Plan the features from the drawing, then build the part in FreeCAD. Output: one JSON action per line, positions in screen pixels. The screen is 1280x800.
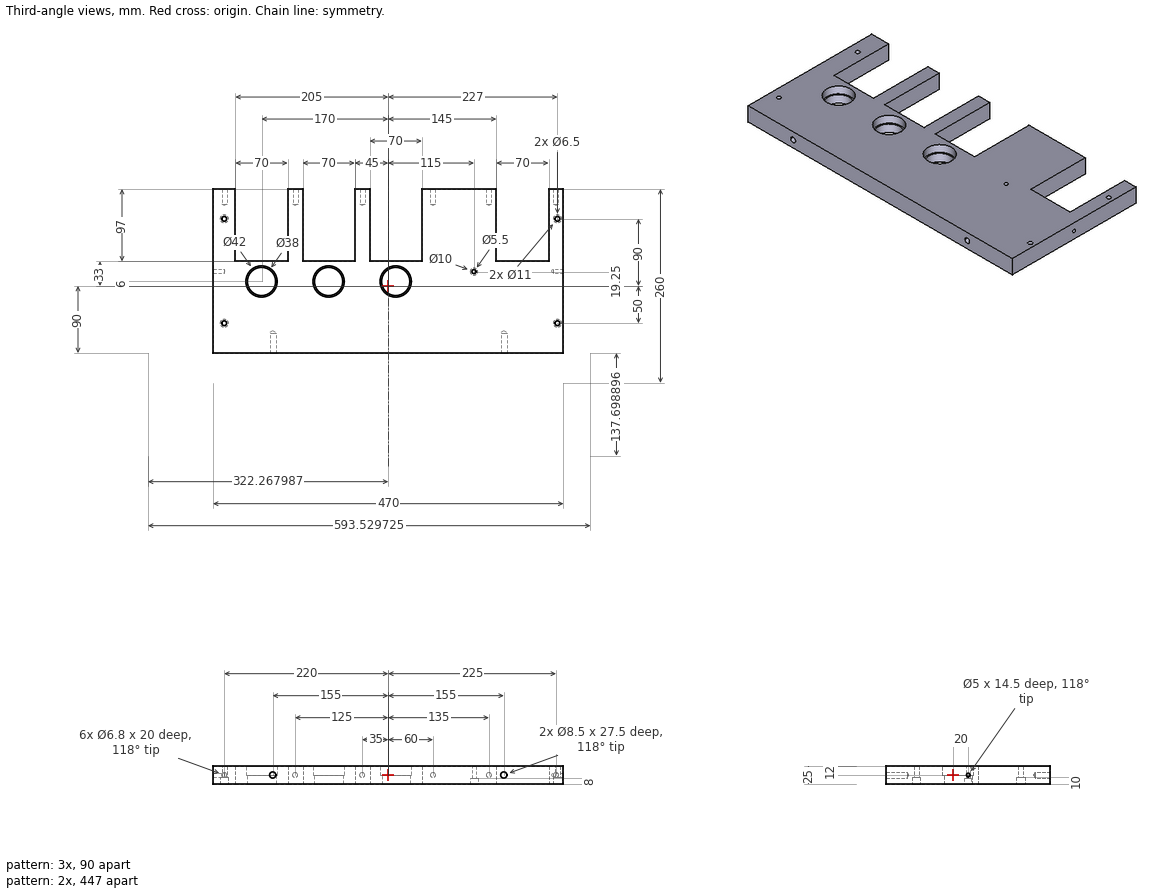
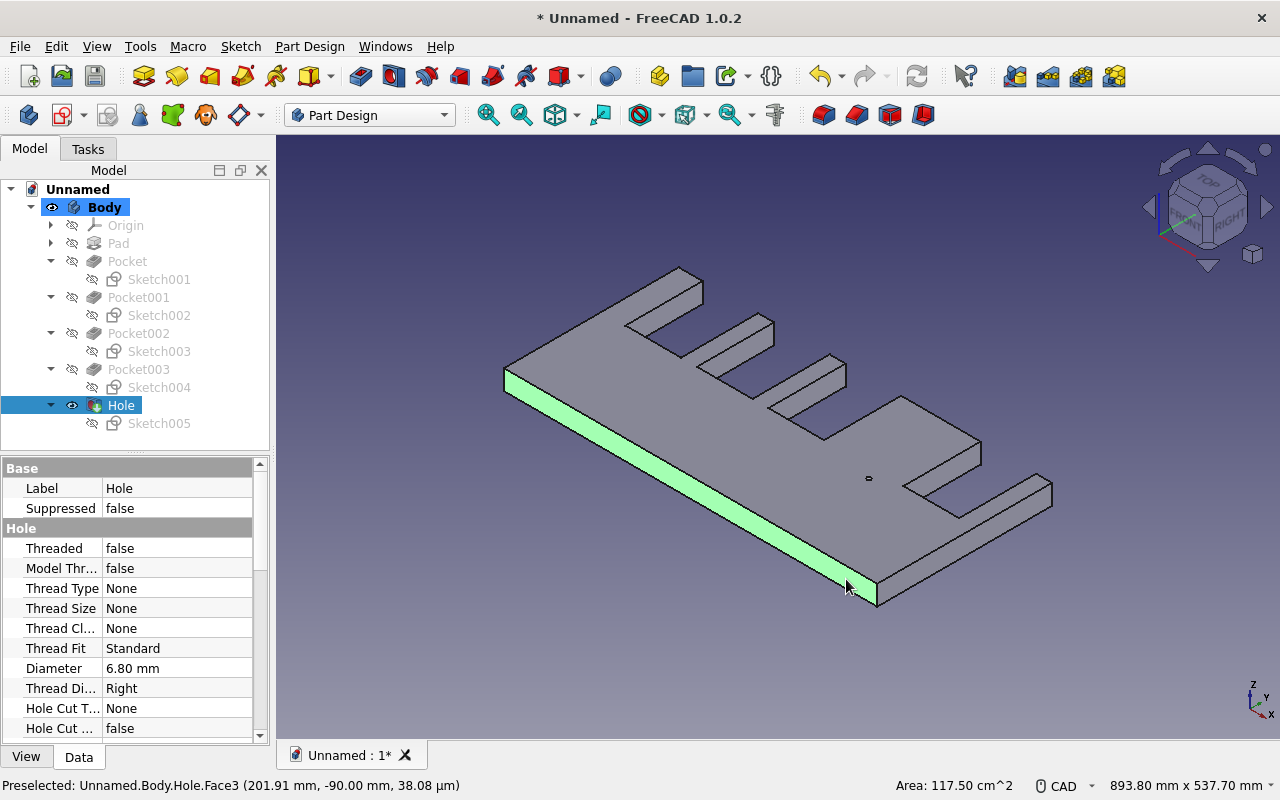
{"action": "left_click", "coordinate": [62, 116]}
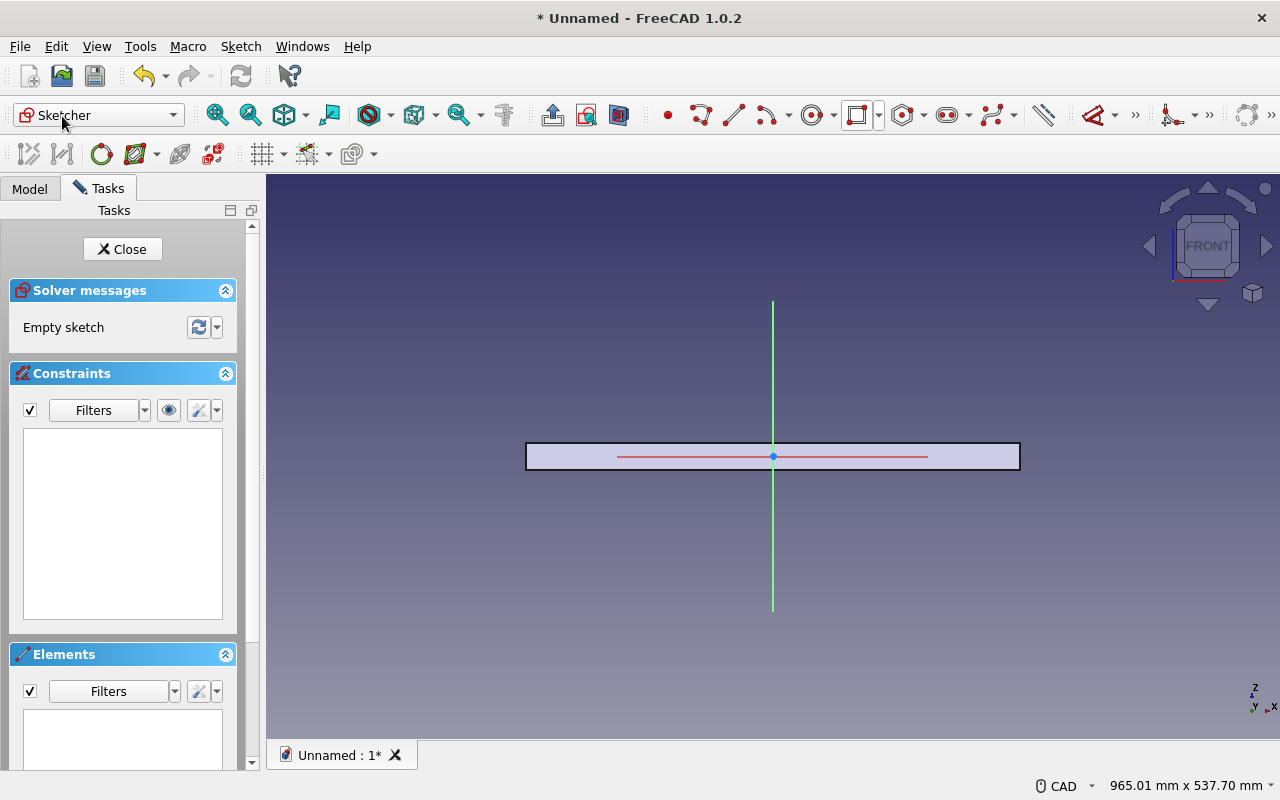
{"action": "scroll", "coordinate": [856, 457], "scroll_direction": "up", "scroll_amount": 3}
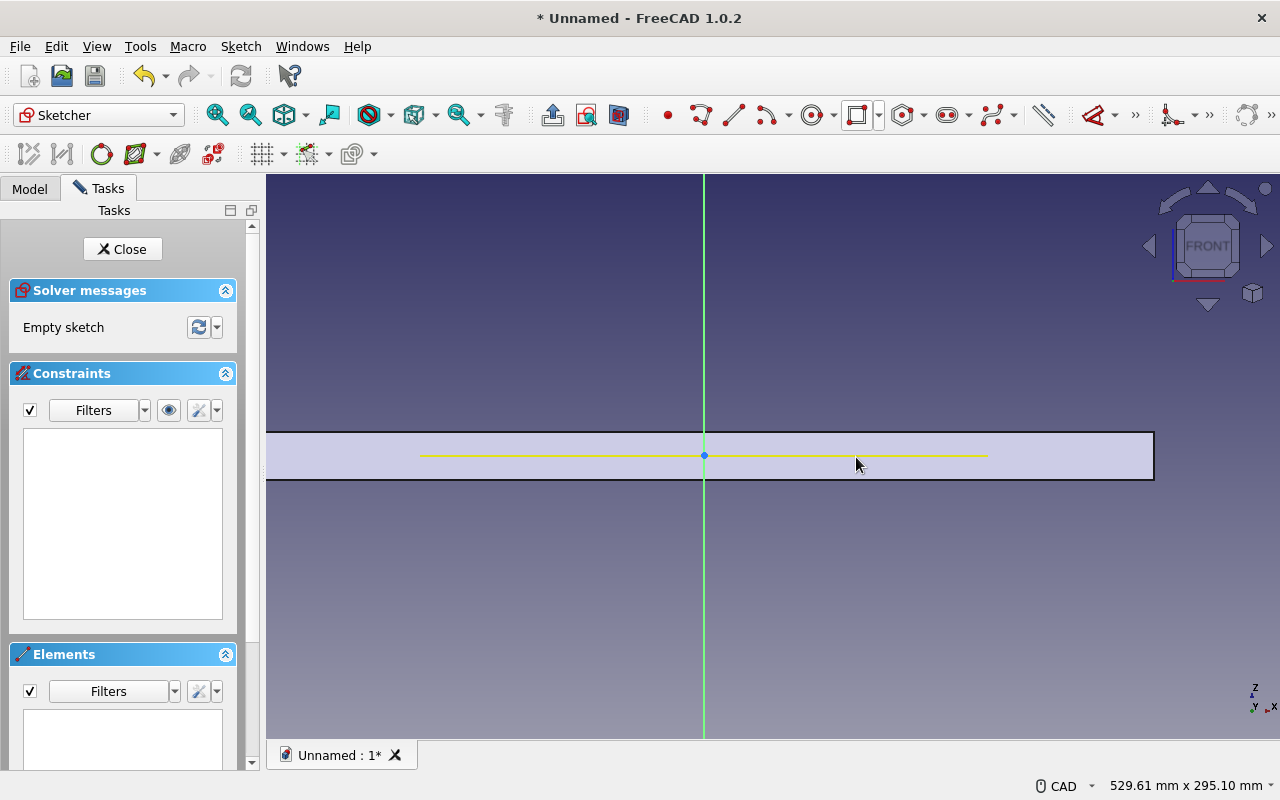
{"action": "left_click", "coordinate": [812, 116]}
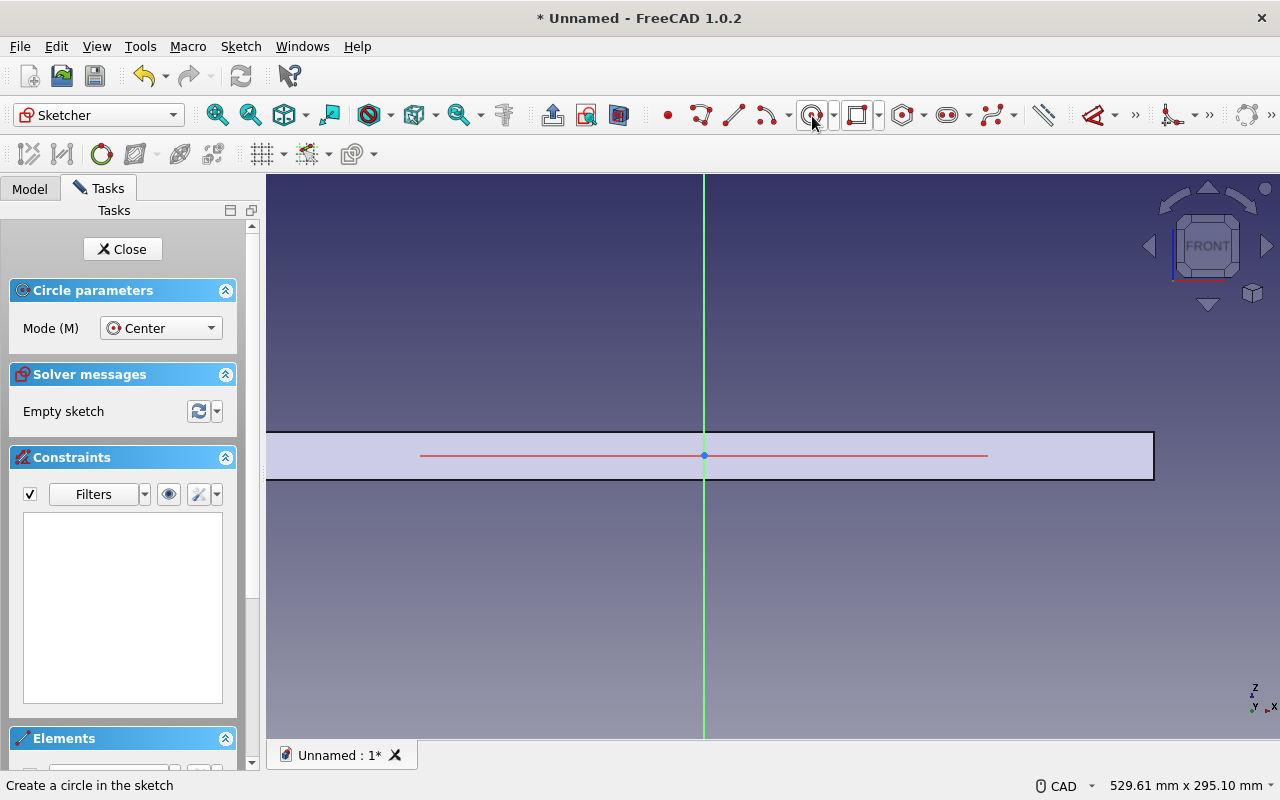
{"action": "scroll", "coordinate": [1001, 456], "scroll_direction": "up", "scroll_amount": 6}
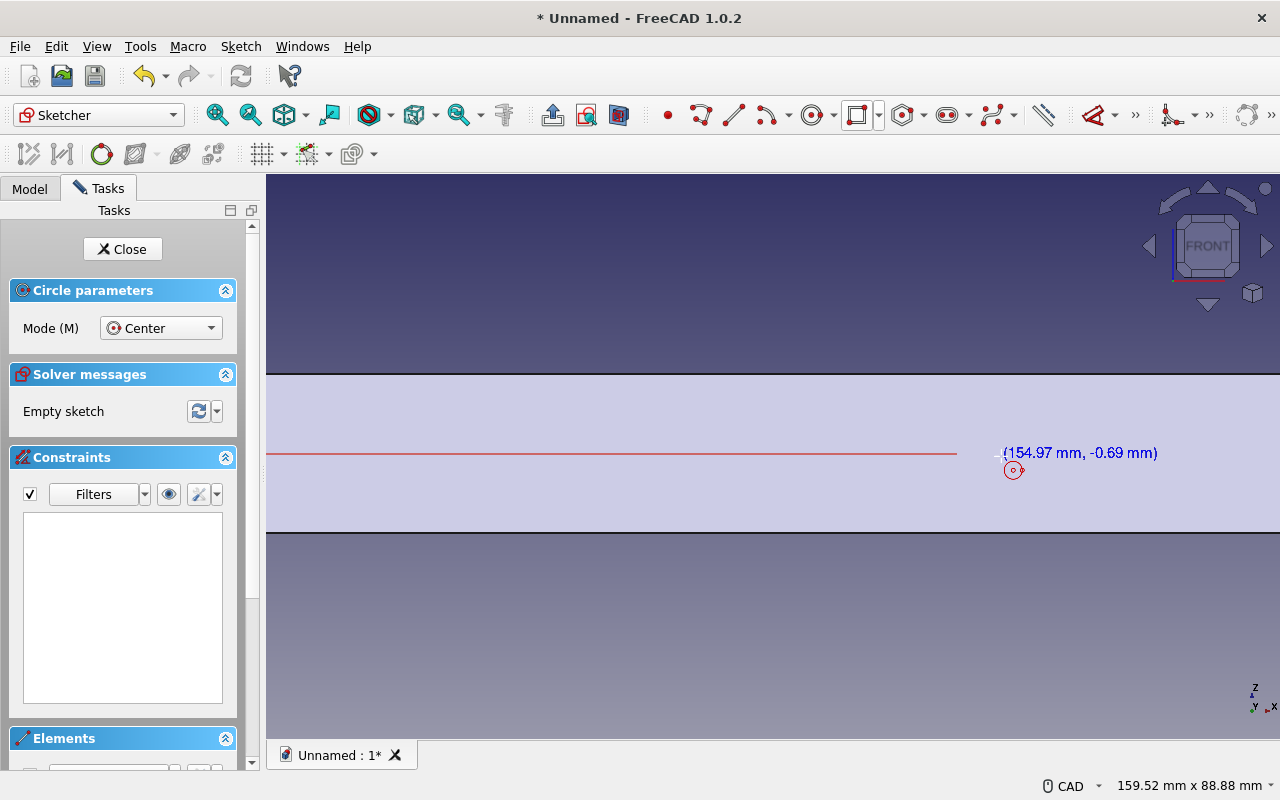
{"action": "left_click", "coordinate": [999, 454]}
{"action": "mouse_move", "coordinate": [1019, 435]}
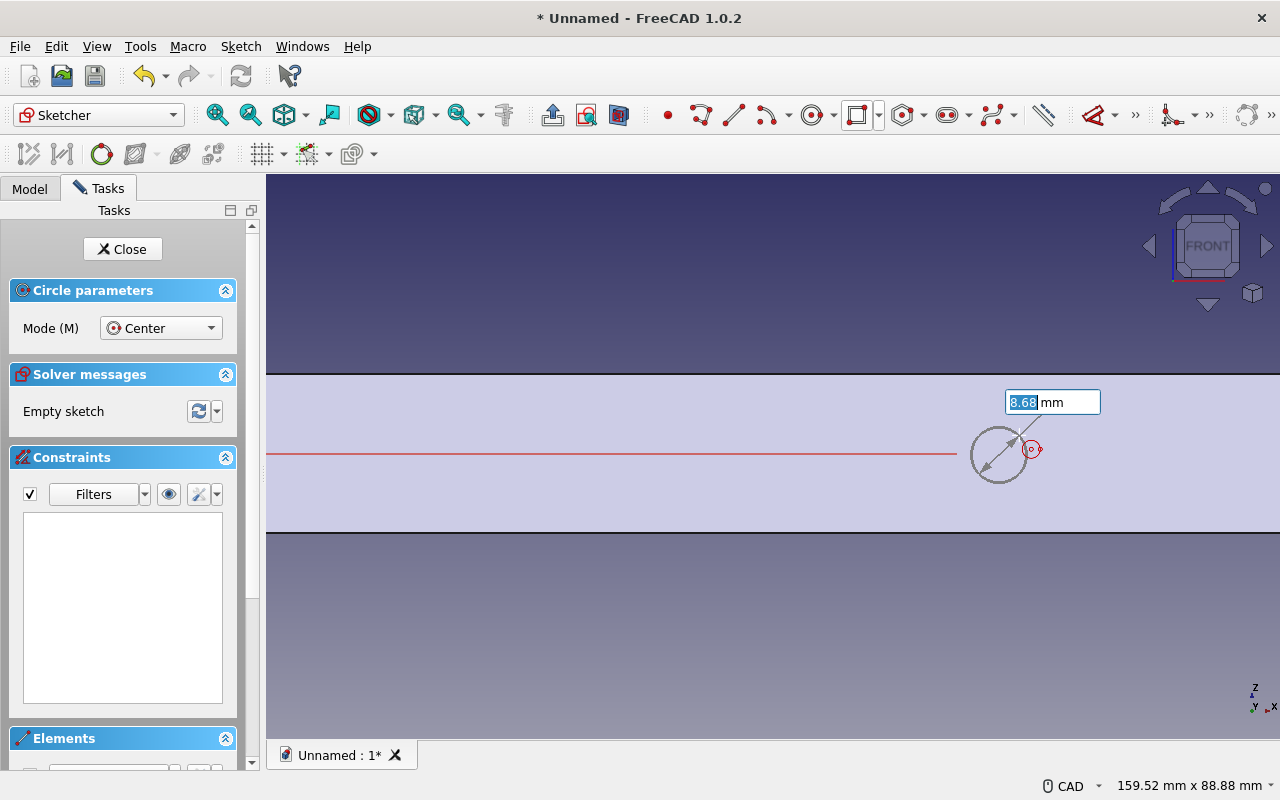
{"action": "type", "text": "8.5"}
{"action": "key", "text": "Return"}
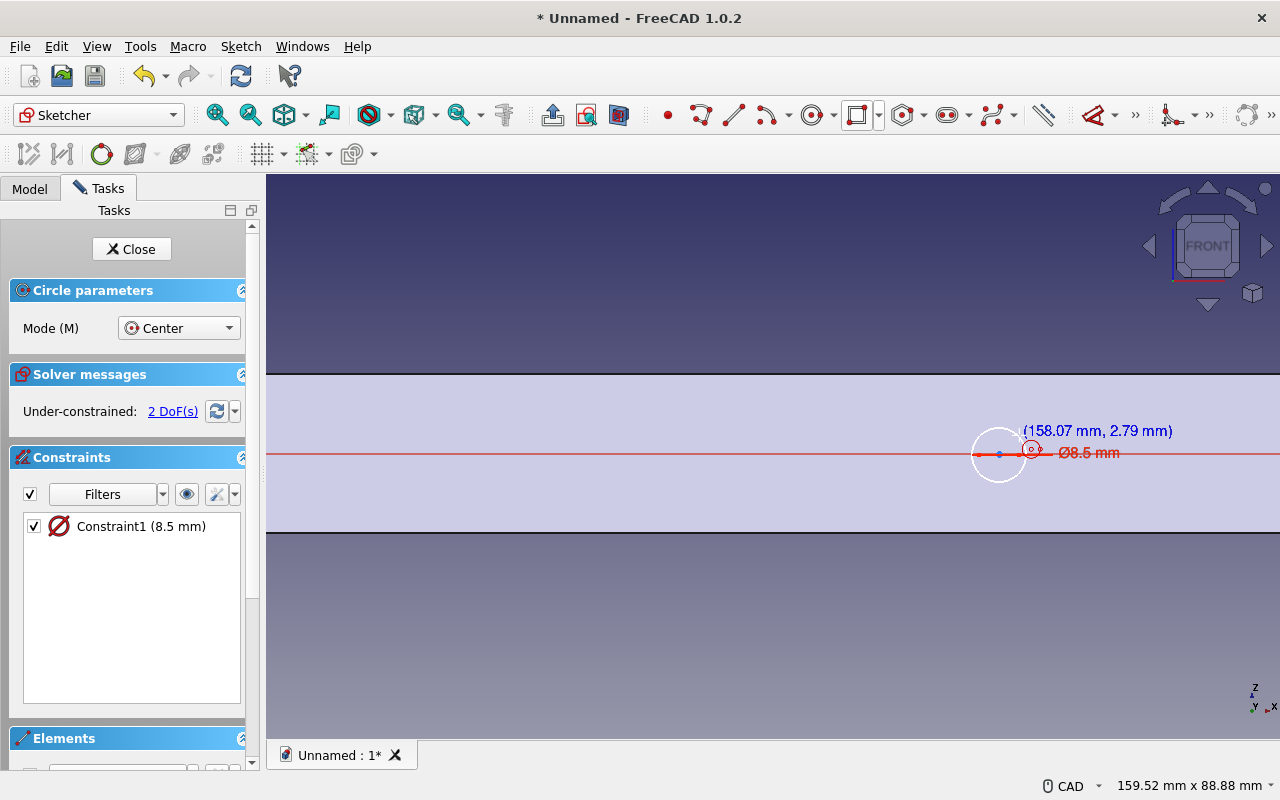
{"action": "scroll", "coordinate": [1002, 458], "scroll_direction": "down", "scroll_amount": 6}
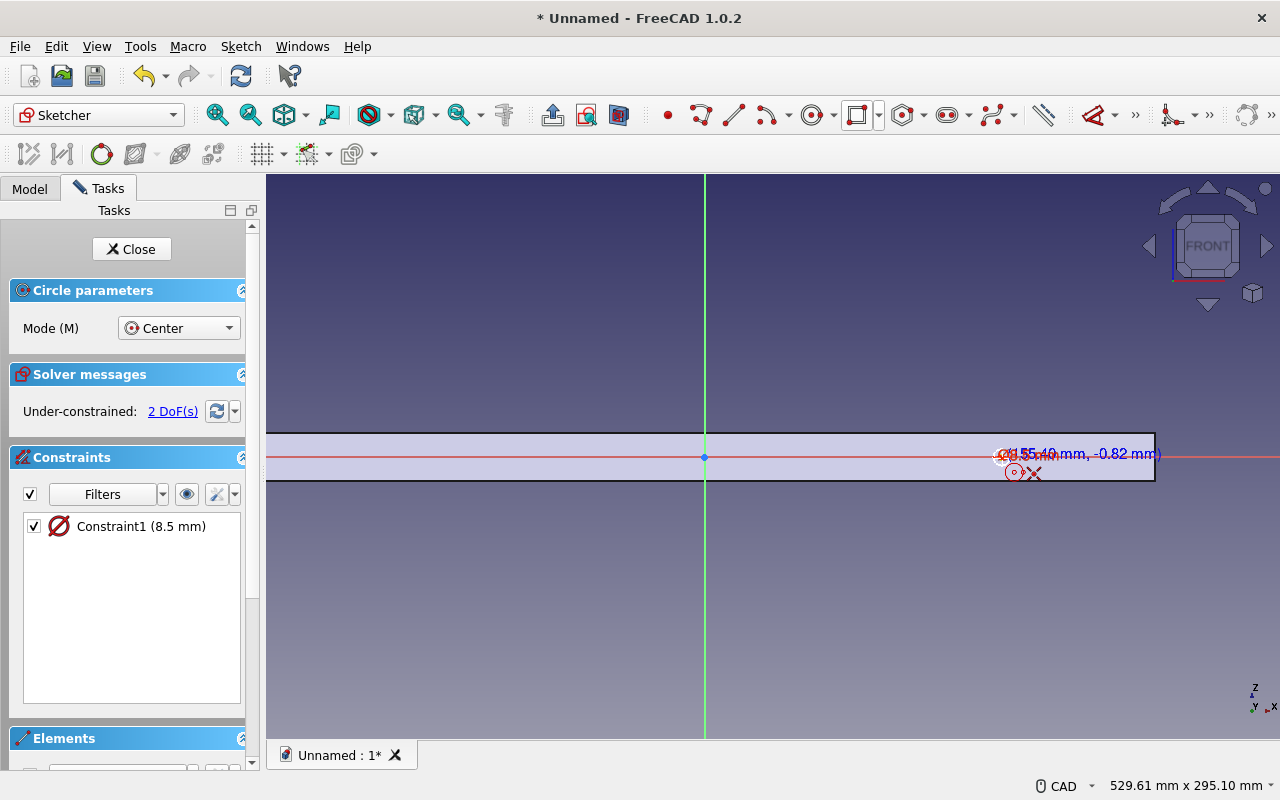
{"action": "scroll", "coordinate": [408, 457], "scroll_direction": "up", "scroll_amount": 6}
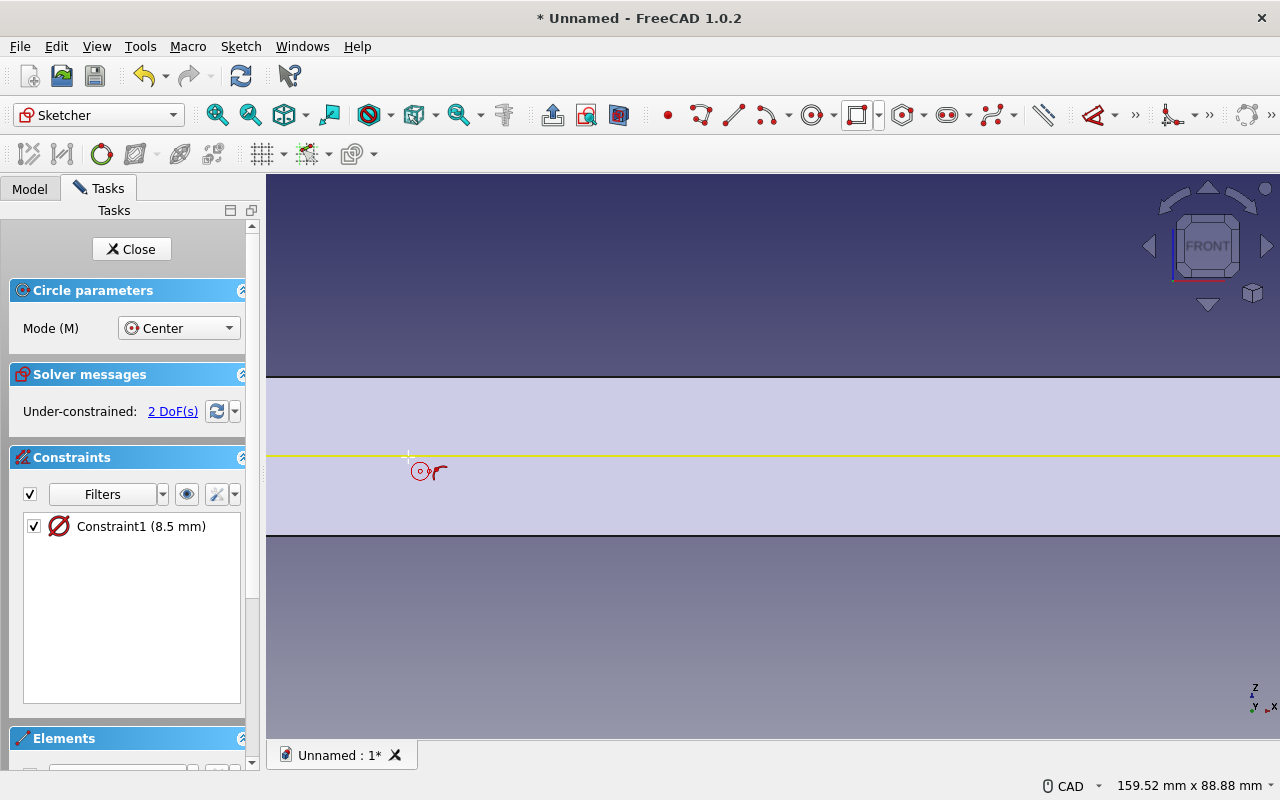
{"action": "left_click", "coordinate": [408, 456]}
{"action": "mouse_move", "coordinate": [428, 437]}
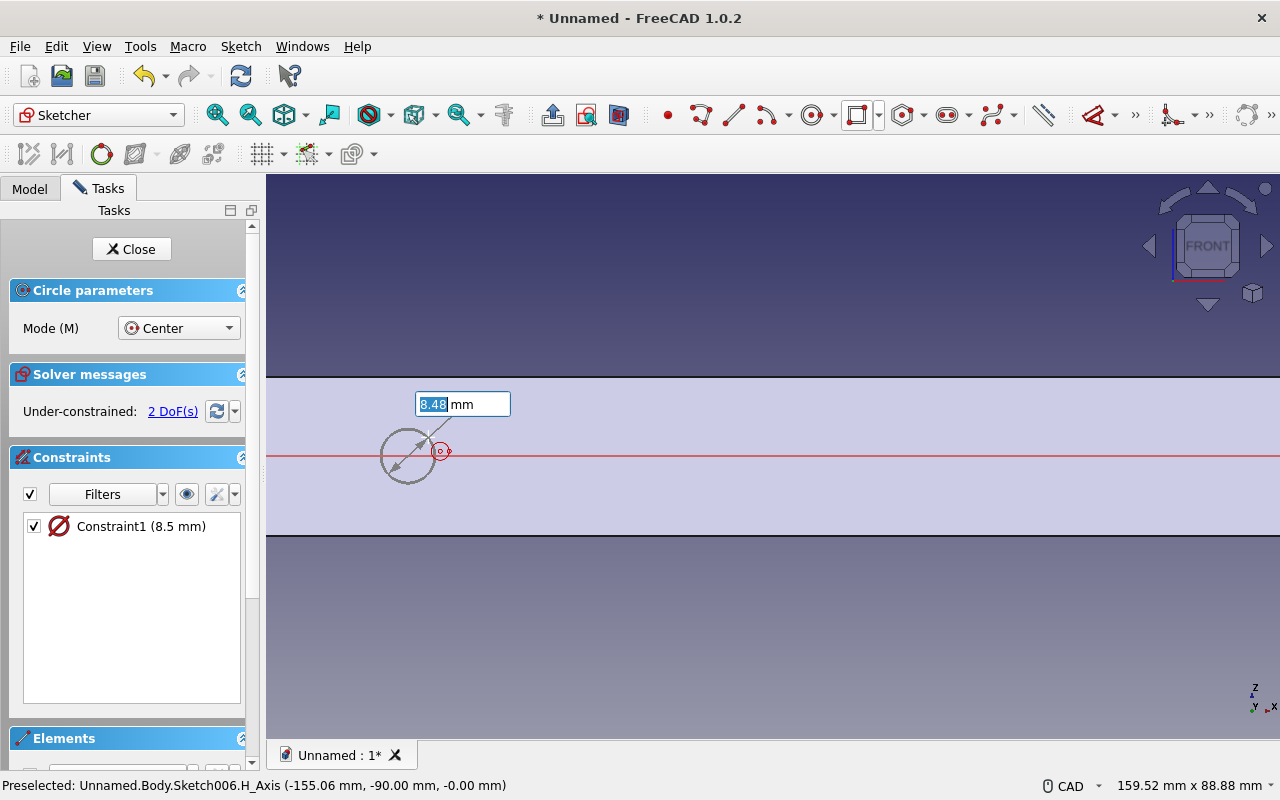
{"action": "type", "text": "8.5"}
{"action": "key", "text": "Return"}
{"action": "key", "text": "Escape"}